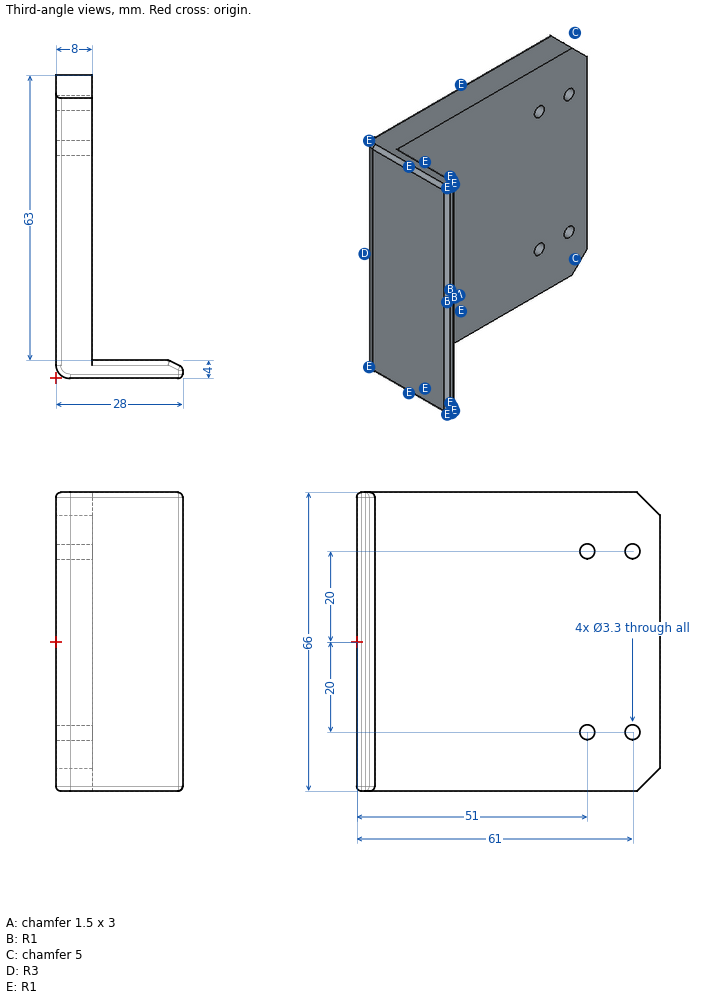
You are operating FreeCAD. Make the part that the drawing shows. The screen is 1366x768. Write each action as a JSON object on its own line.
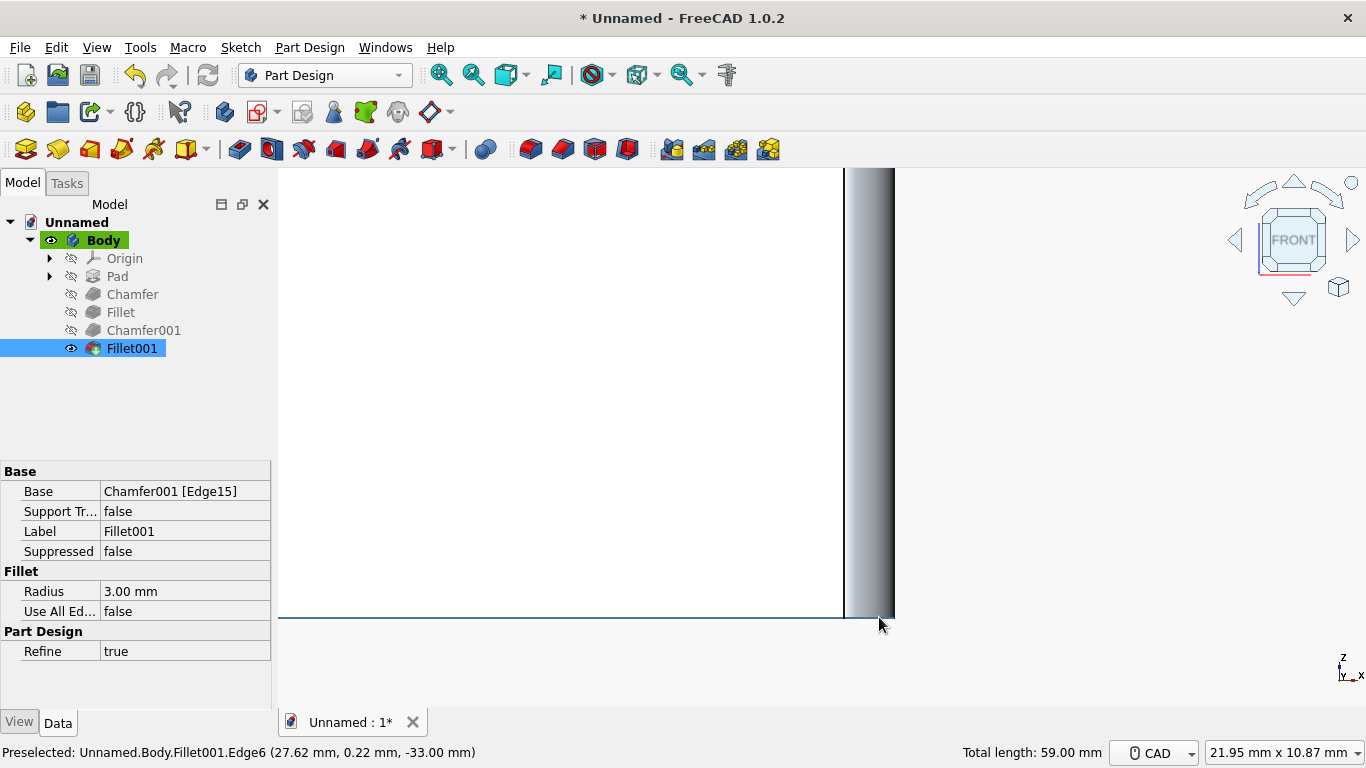
{"action": "left_click", "coordinate": [442, 76]}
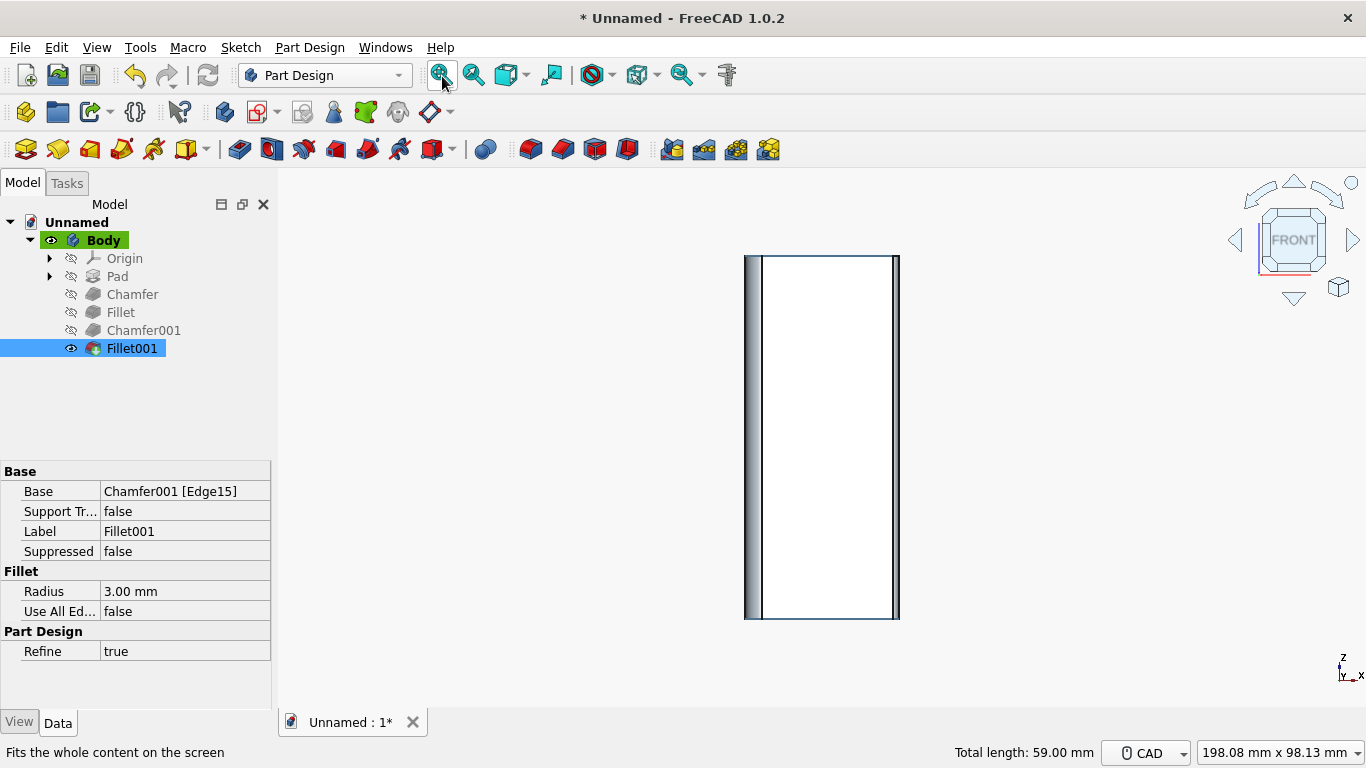
{"action": "key", "text": "0"}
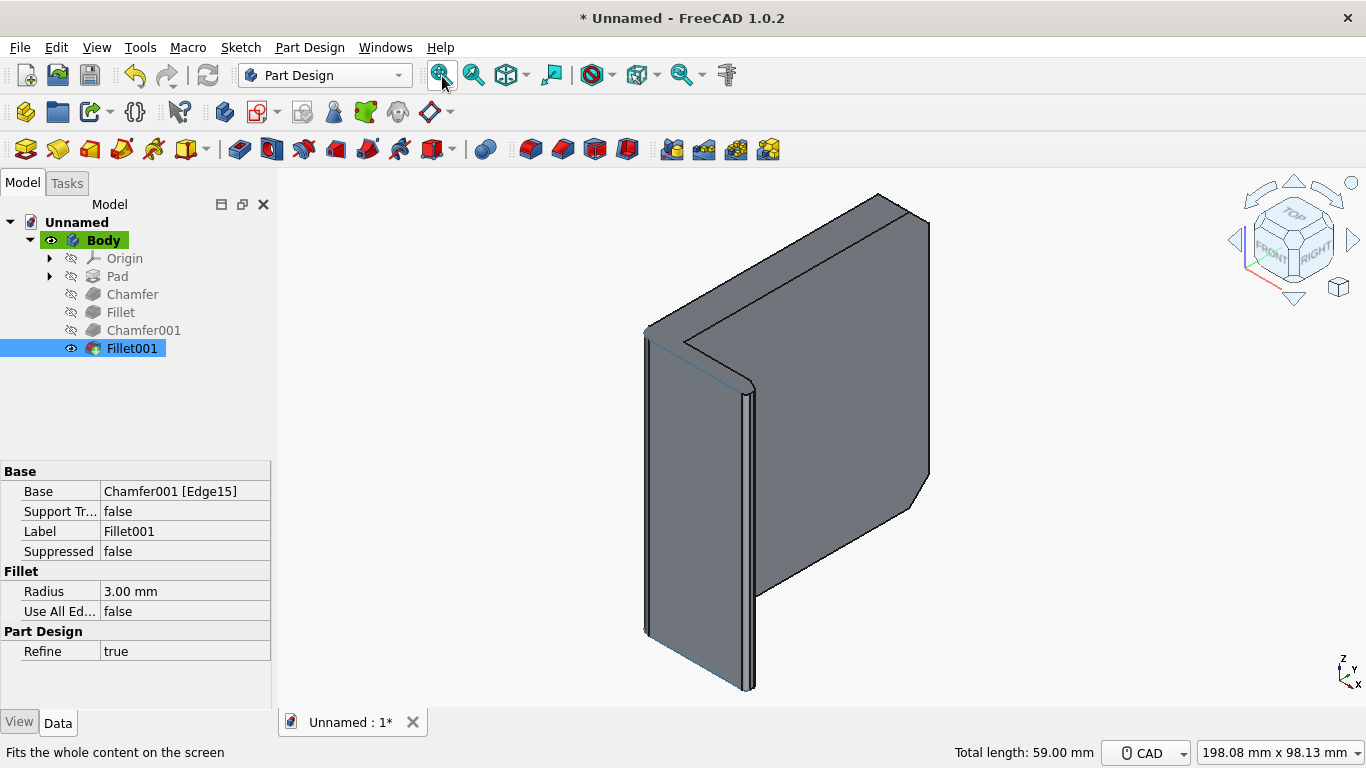
{"action": "left_click", "coordinate": [746, 394], "text": "ctrl"}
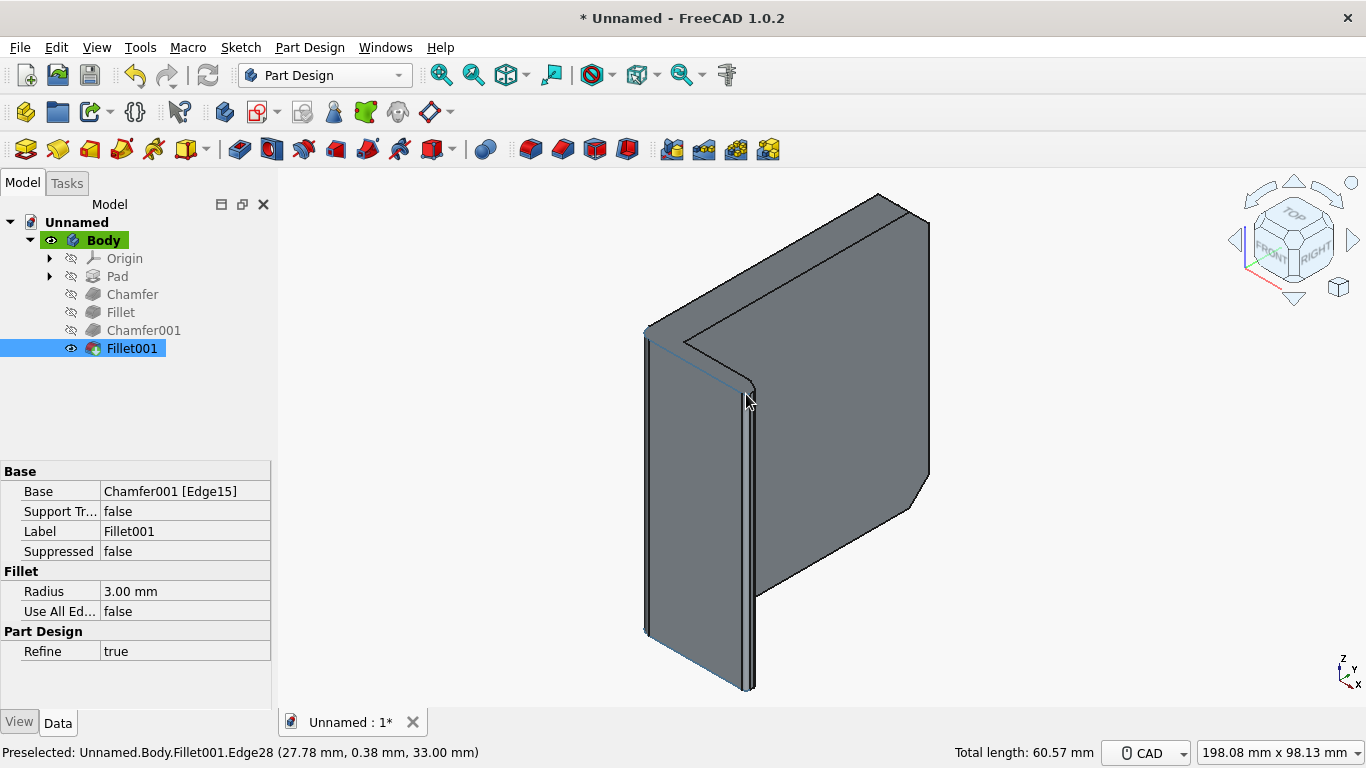
{"action": "key", "text": "2"}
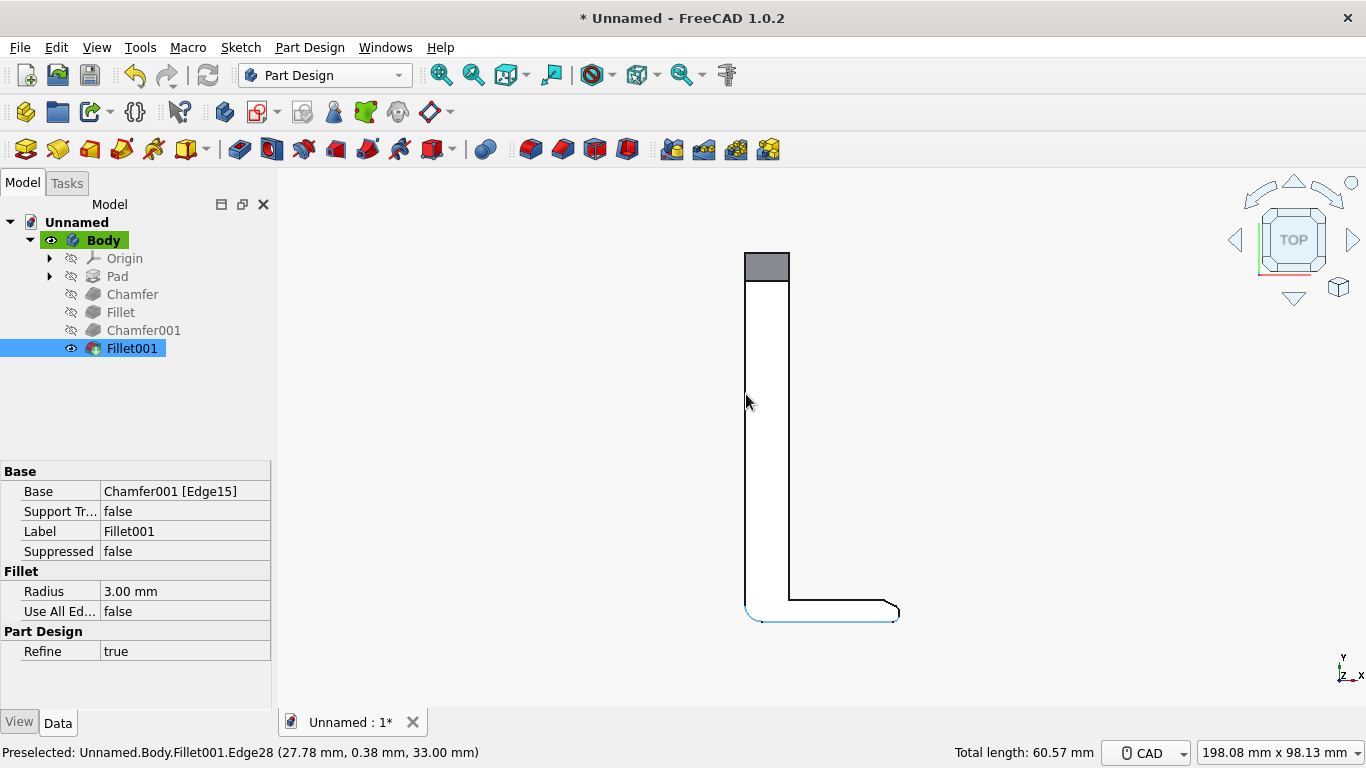
{"action": "left_click", "coordinate": [890, 602], "text": "ctrl"}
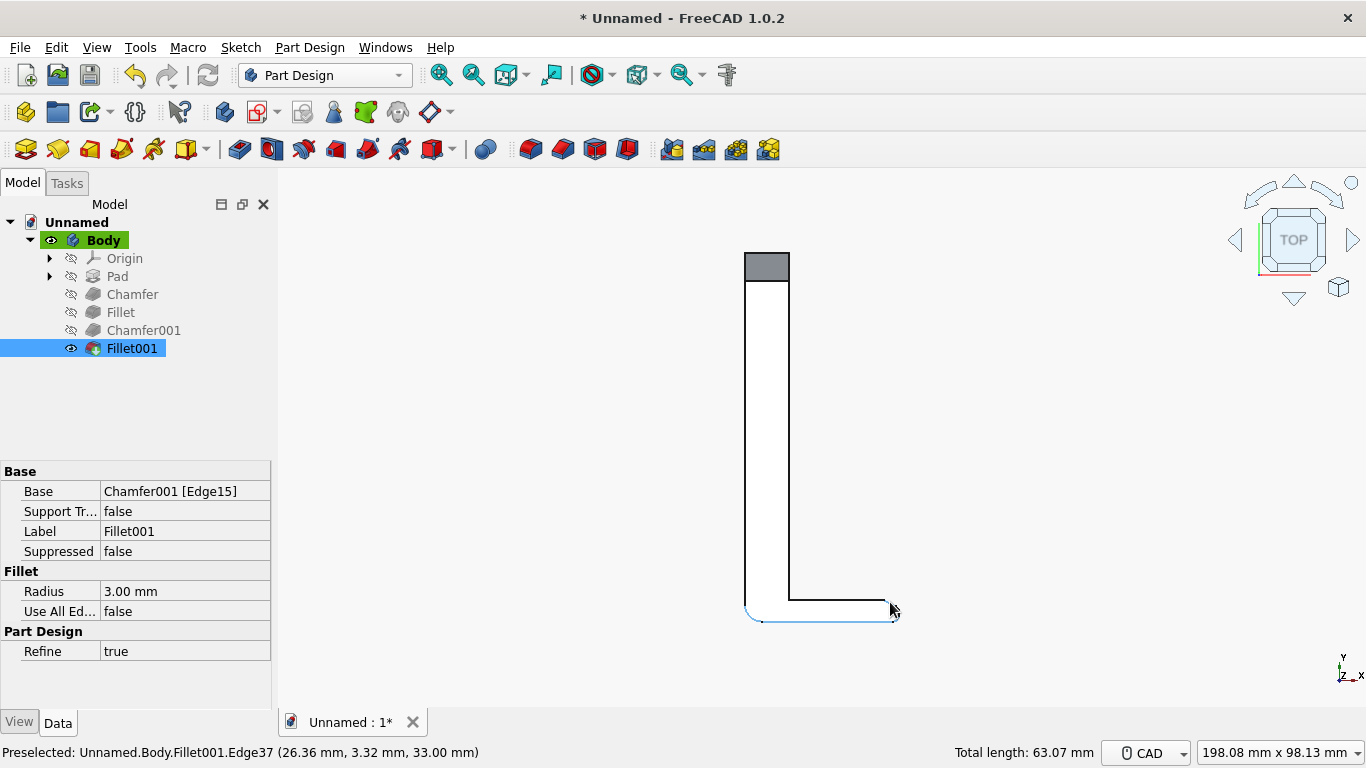
{"action": "left_click", "coordinate": [835, 599], "text": "ctrl"}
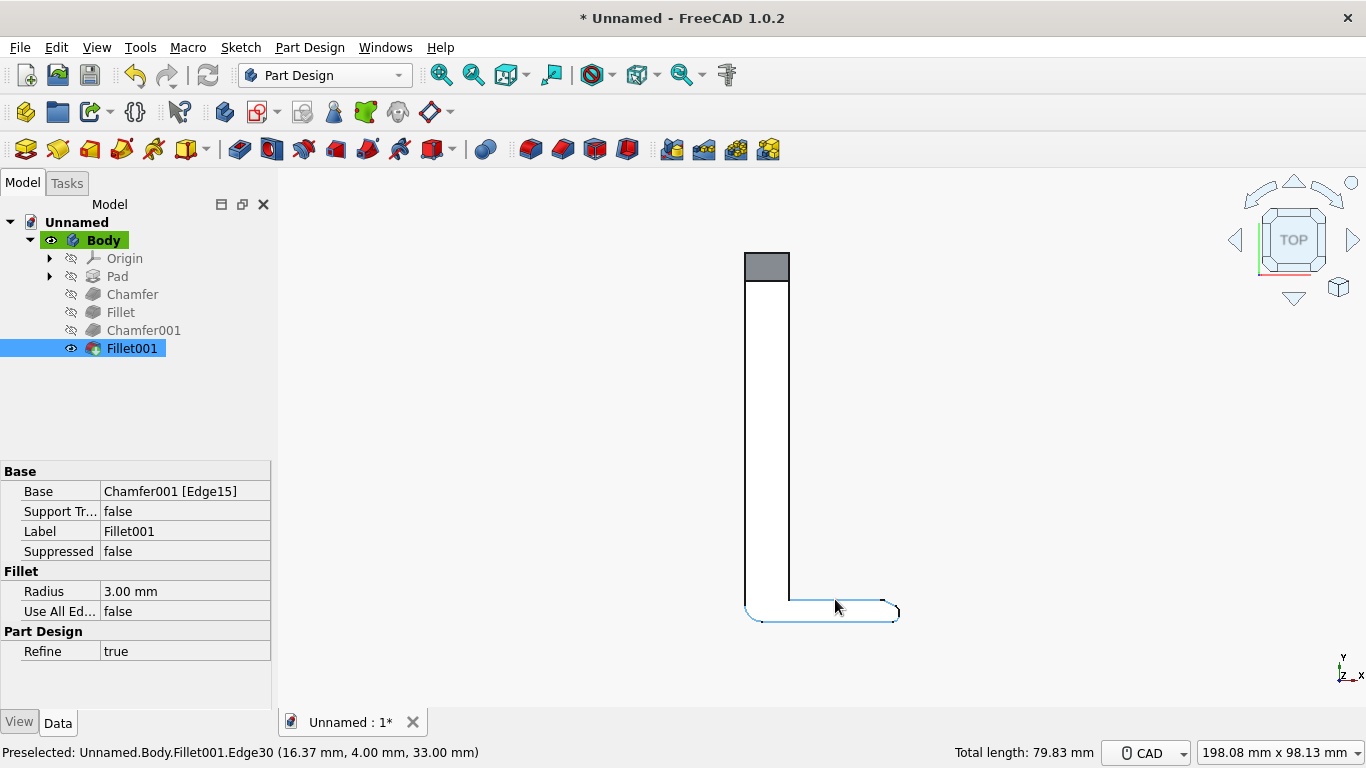
{"action": "left_click", "coordinate": [745, 442], "text": "ctrl"}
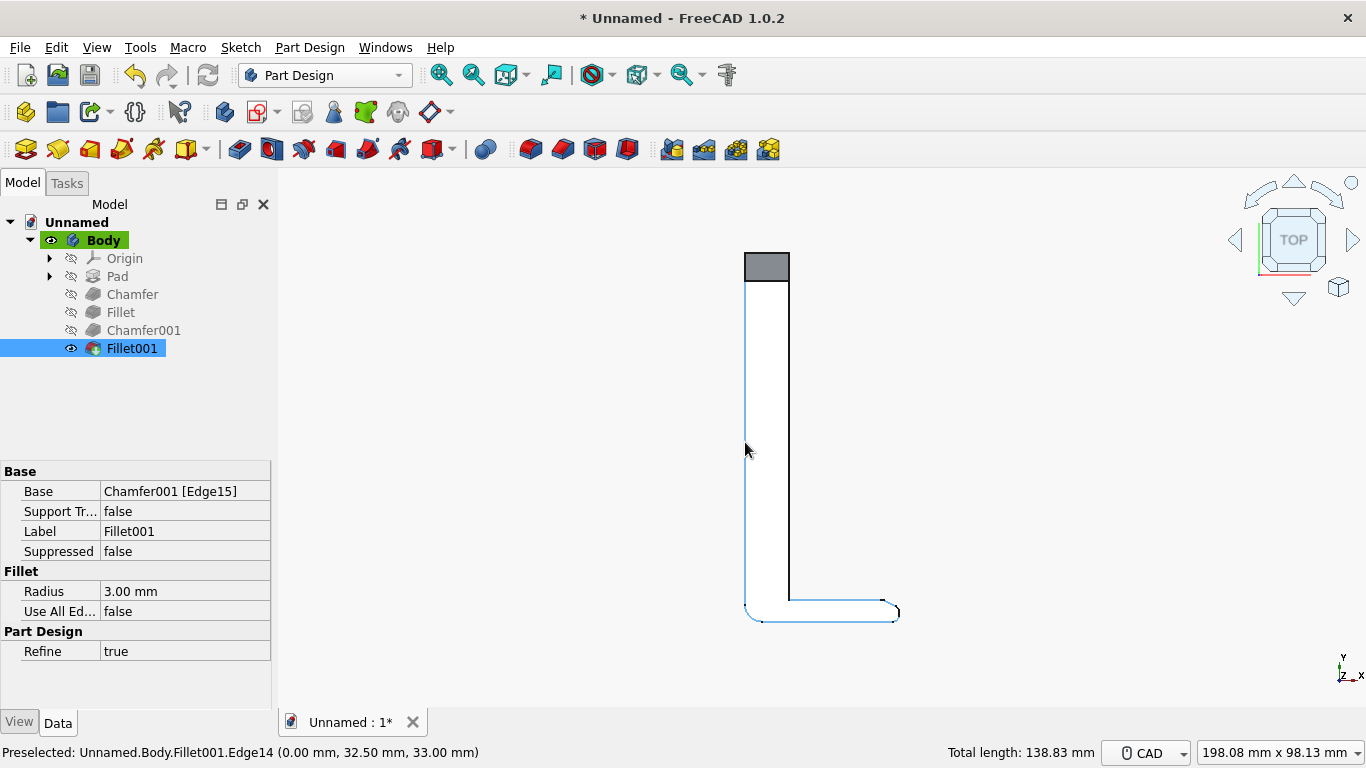
{"action": "scroll", "coordinate": [899, 613], "scroll_direction": "up", "scroll_amount": 11}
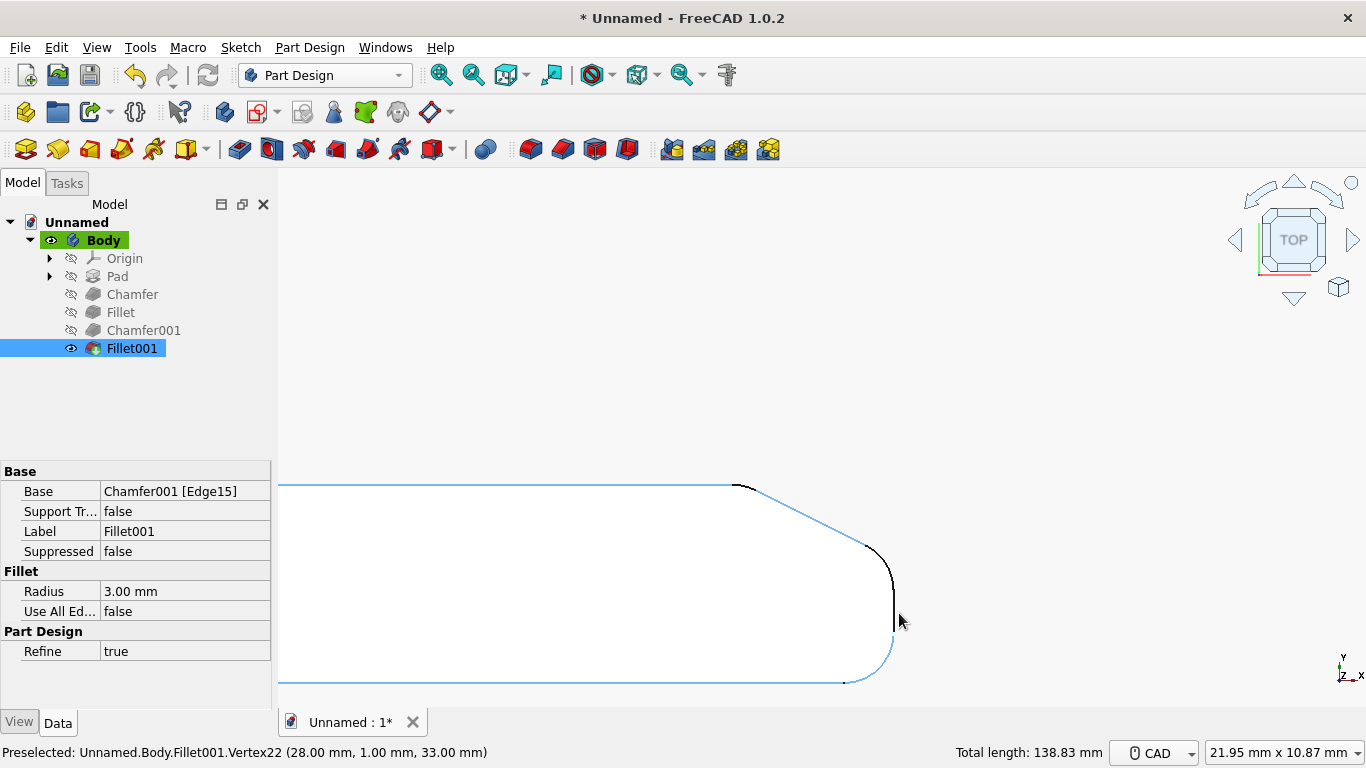
{"action": "left_click", "coordinate": [894, 611], "text": "ctrl"}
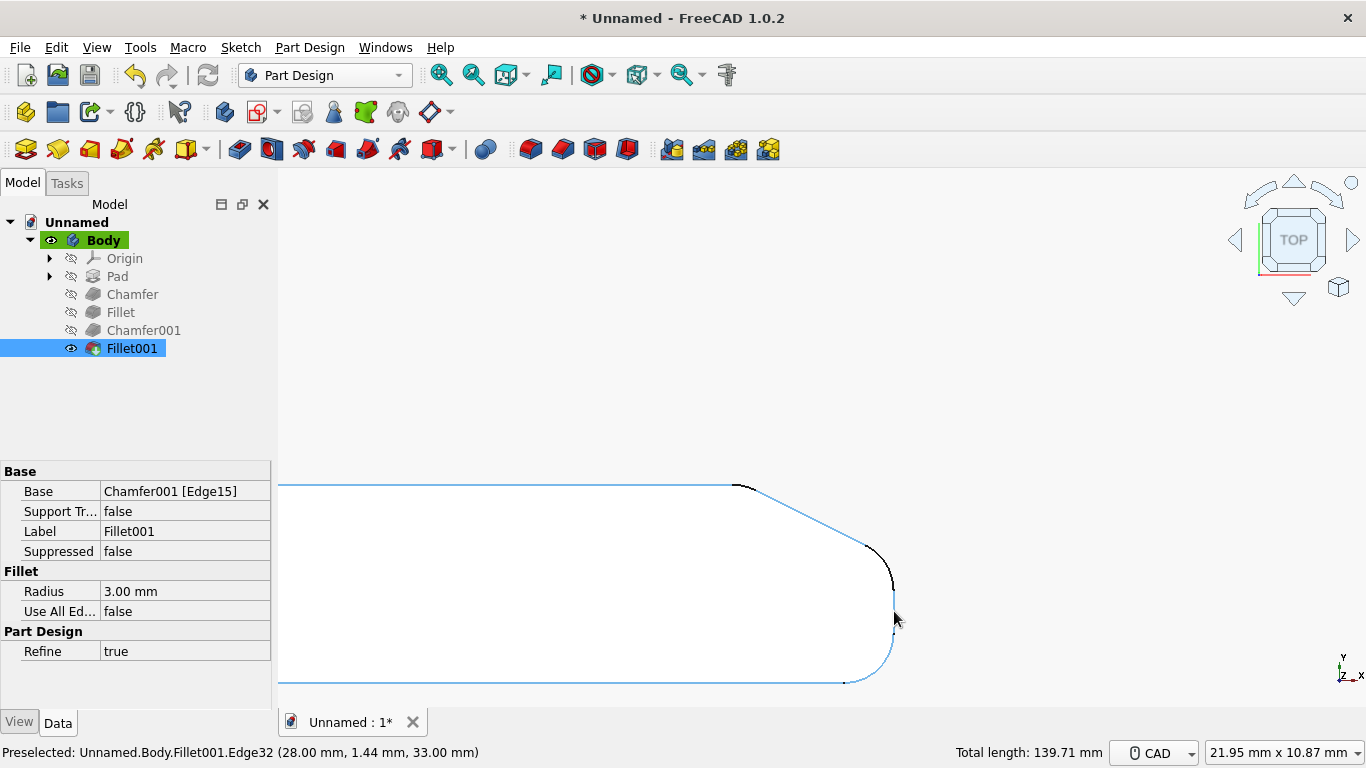
{"action": "left_click", "coordinate": [744, 485], "text": "ctrl"}